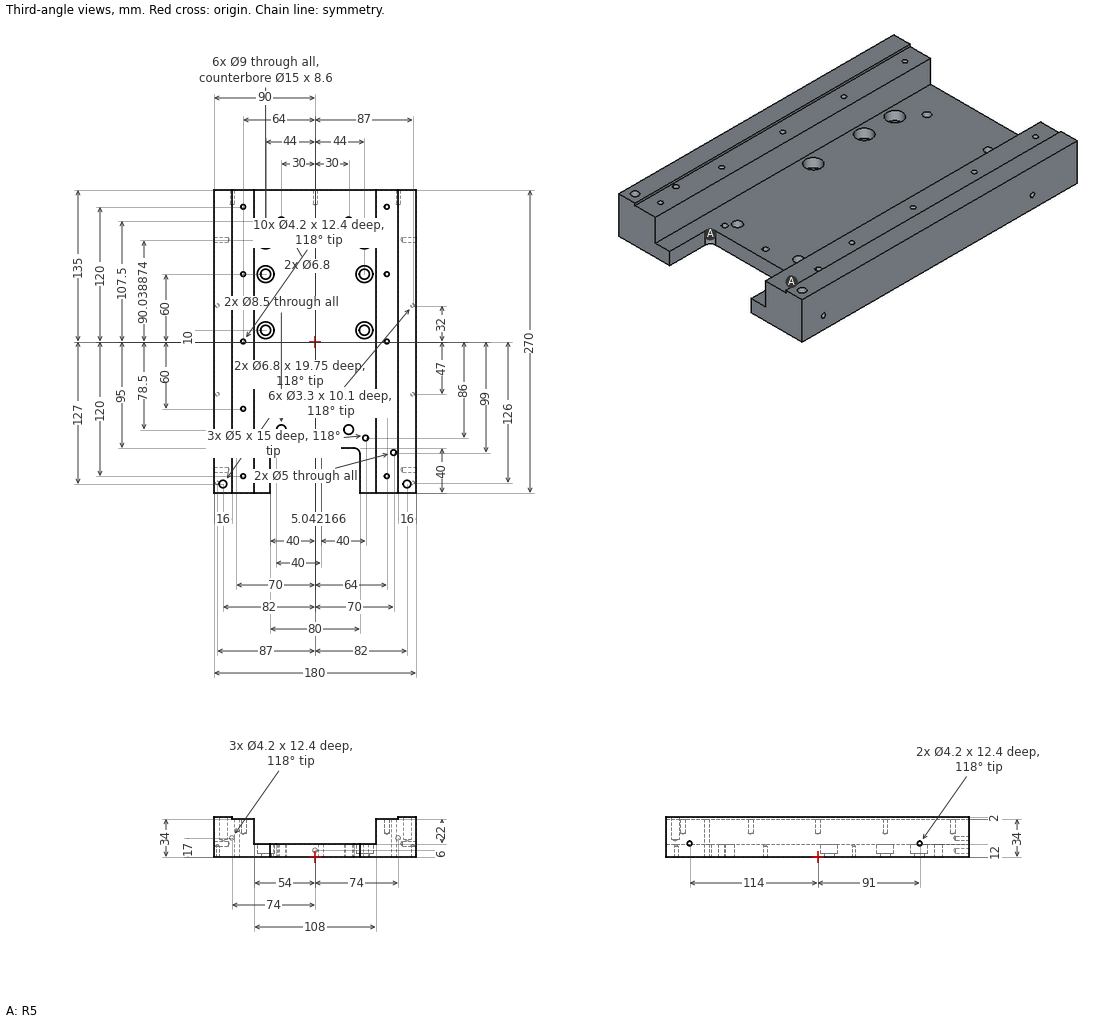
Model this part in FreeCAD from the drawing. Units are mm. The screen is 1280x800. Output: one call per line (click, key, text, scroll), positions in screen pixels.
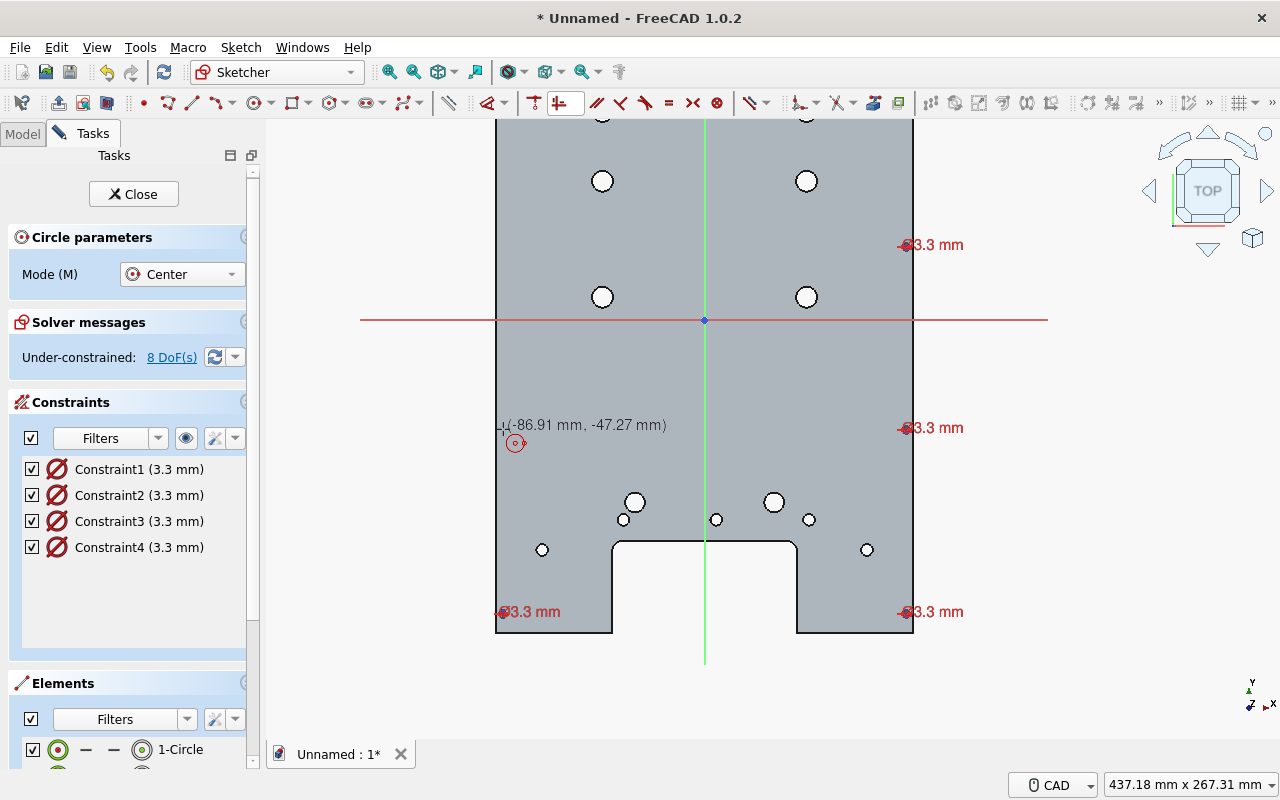
click(503, 429)
move(505, 427)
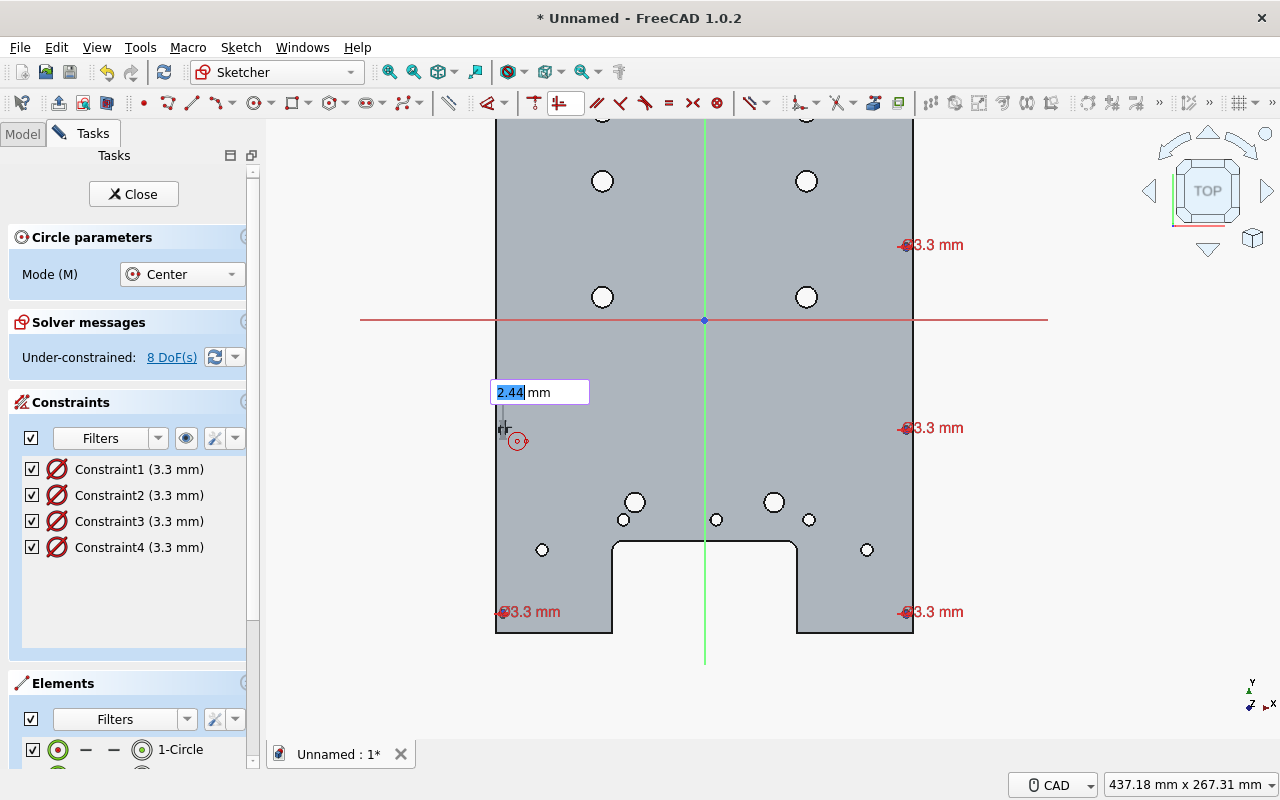
text(3.3)
key(Return)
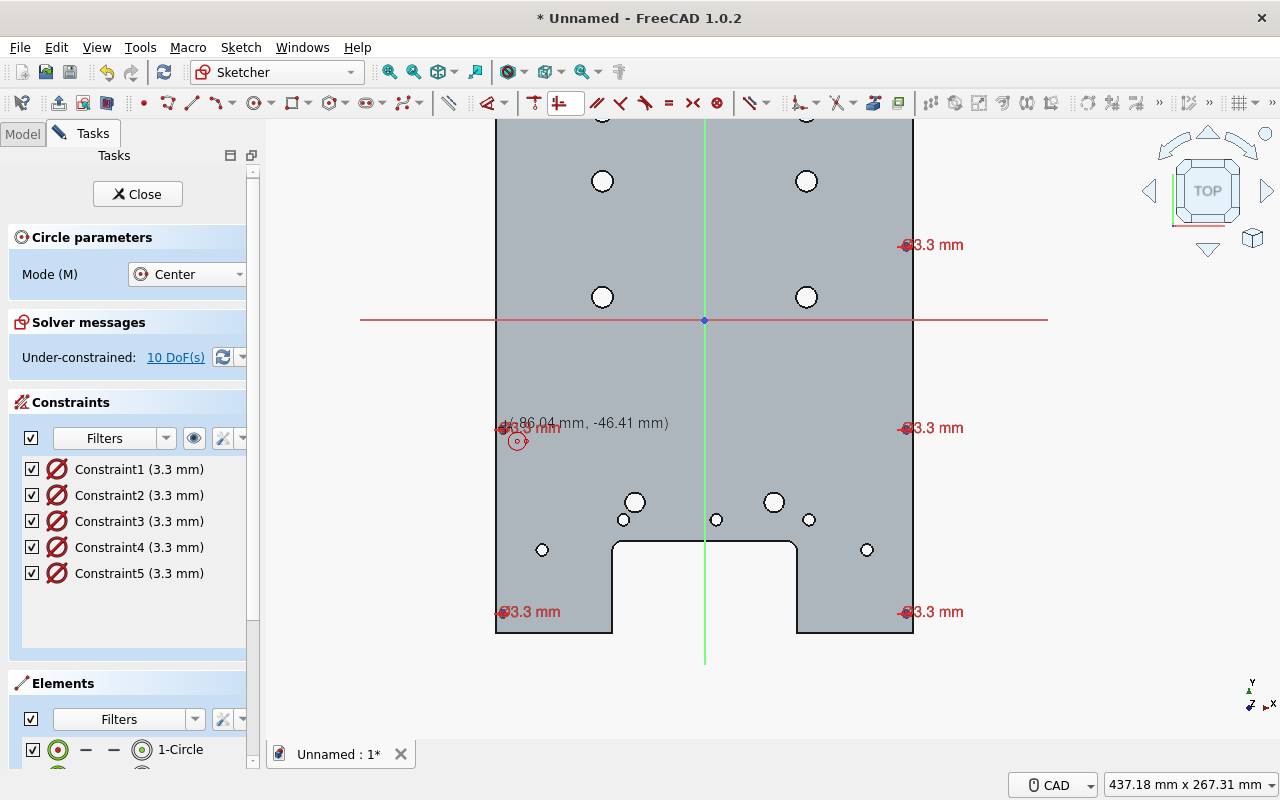
scroll(503, 246, up, 9)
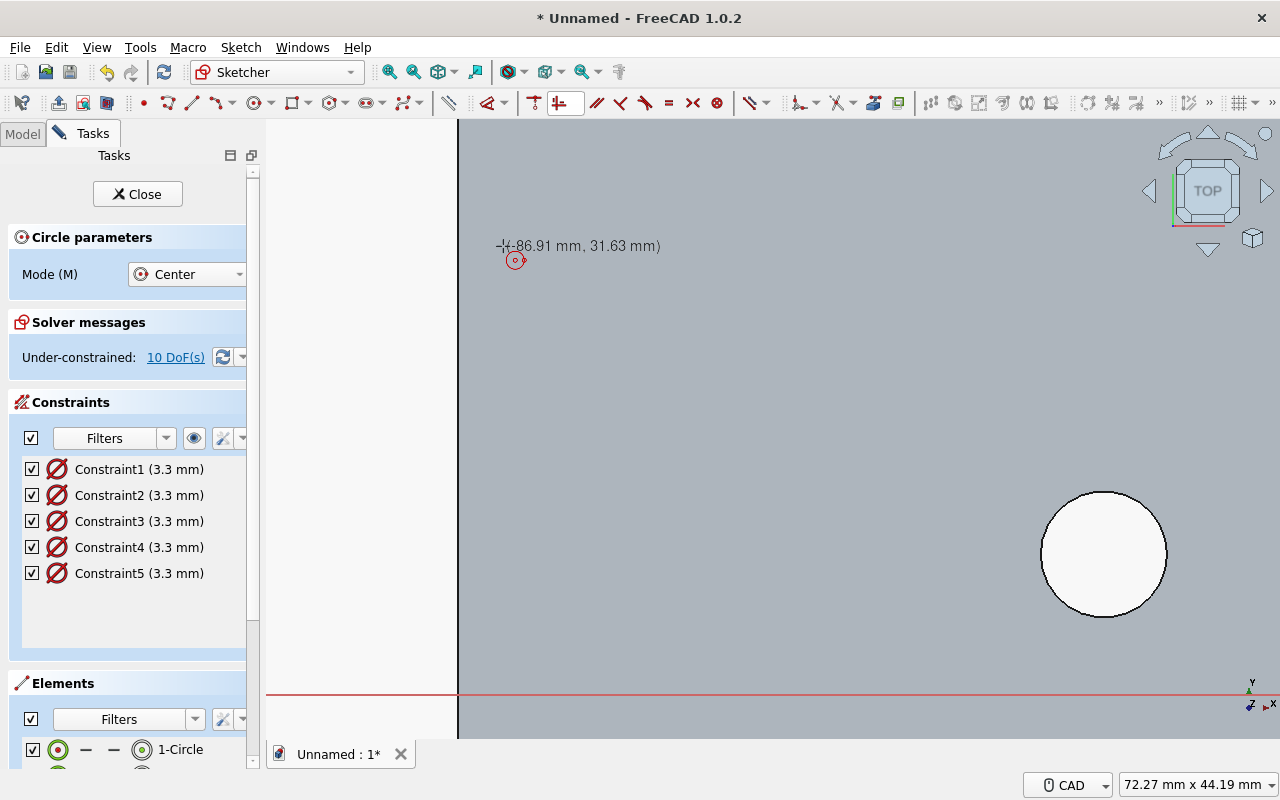
scroll(503, 246, down, 9)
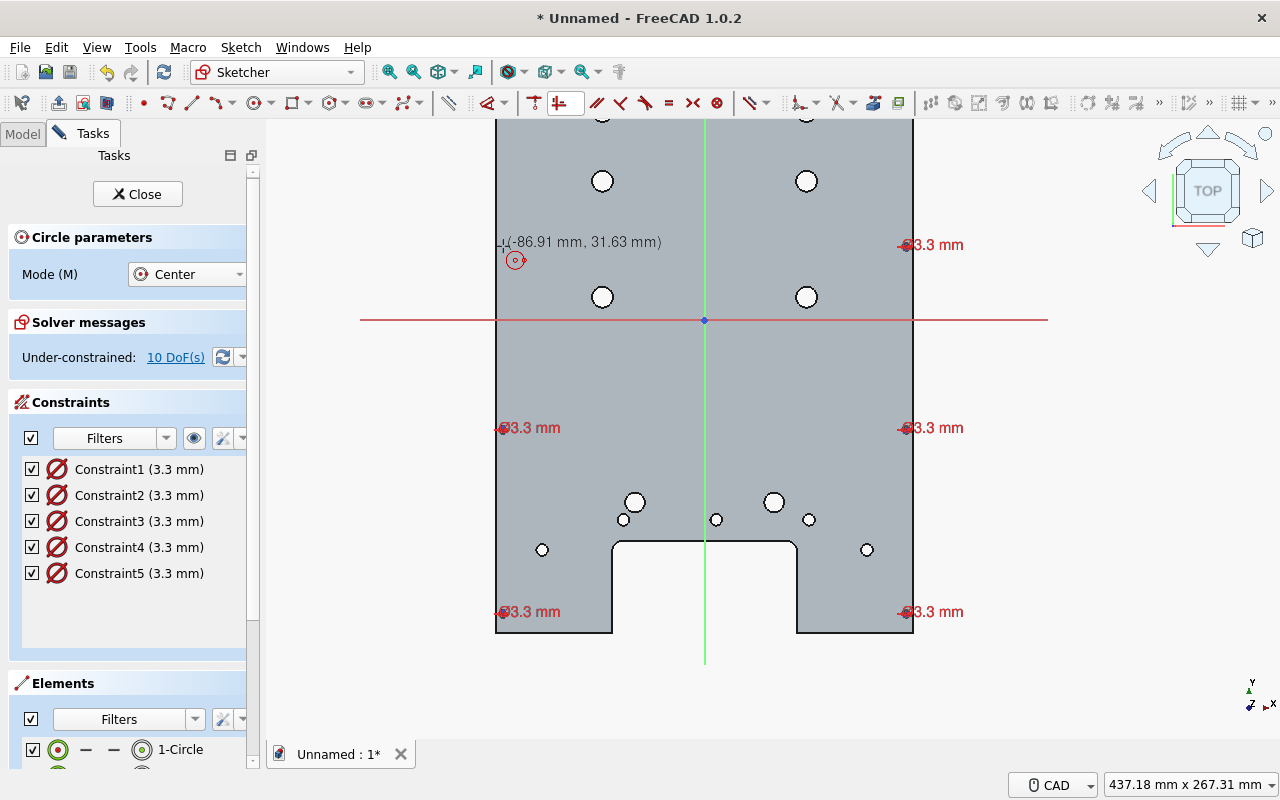
click(503, 246)
move(505, 243)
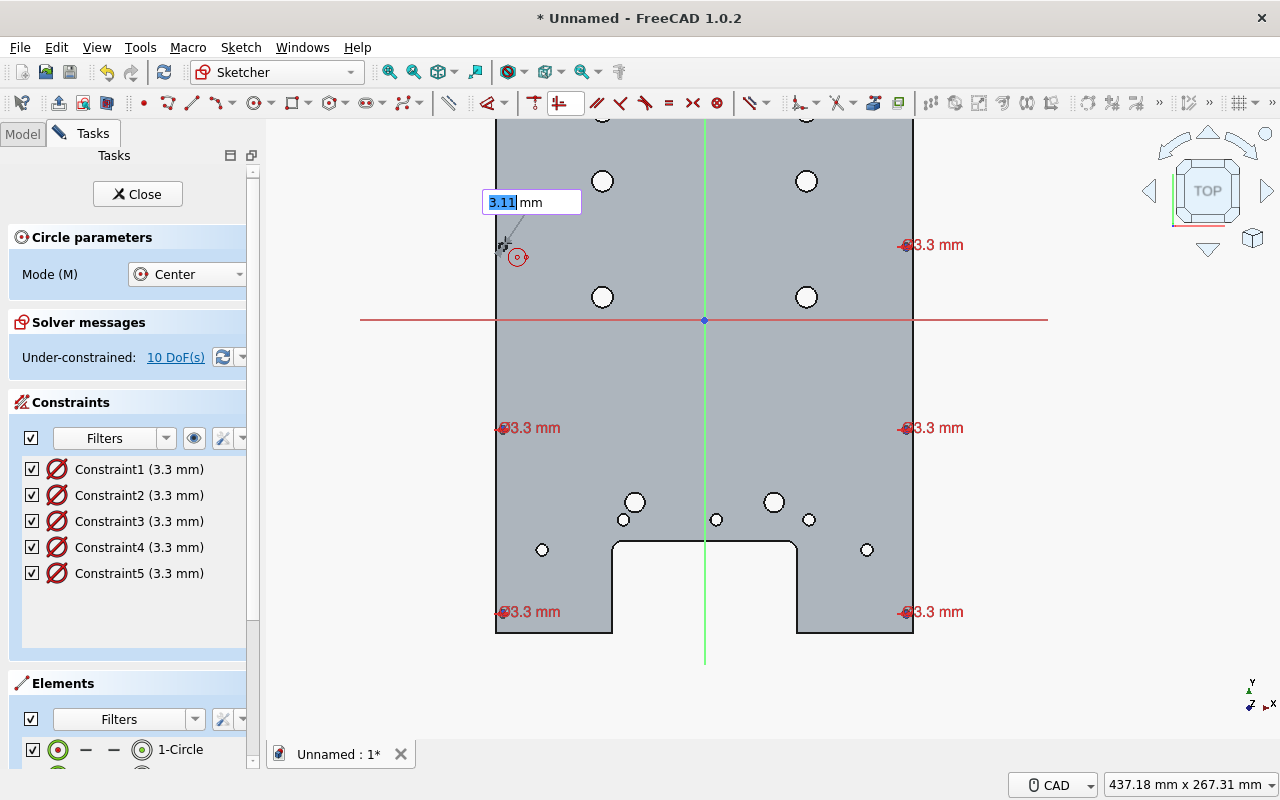
text(3.3)
key(Return)
key(Escape)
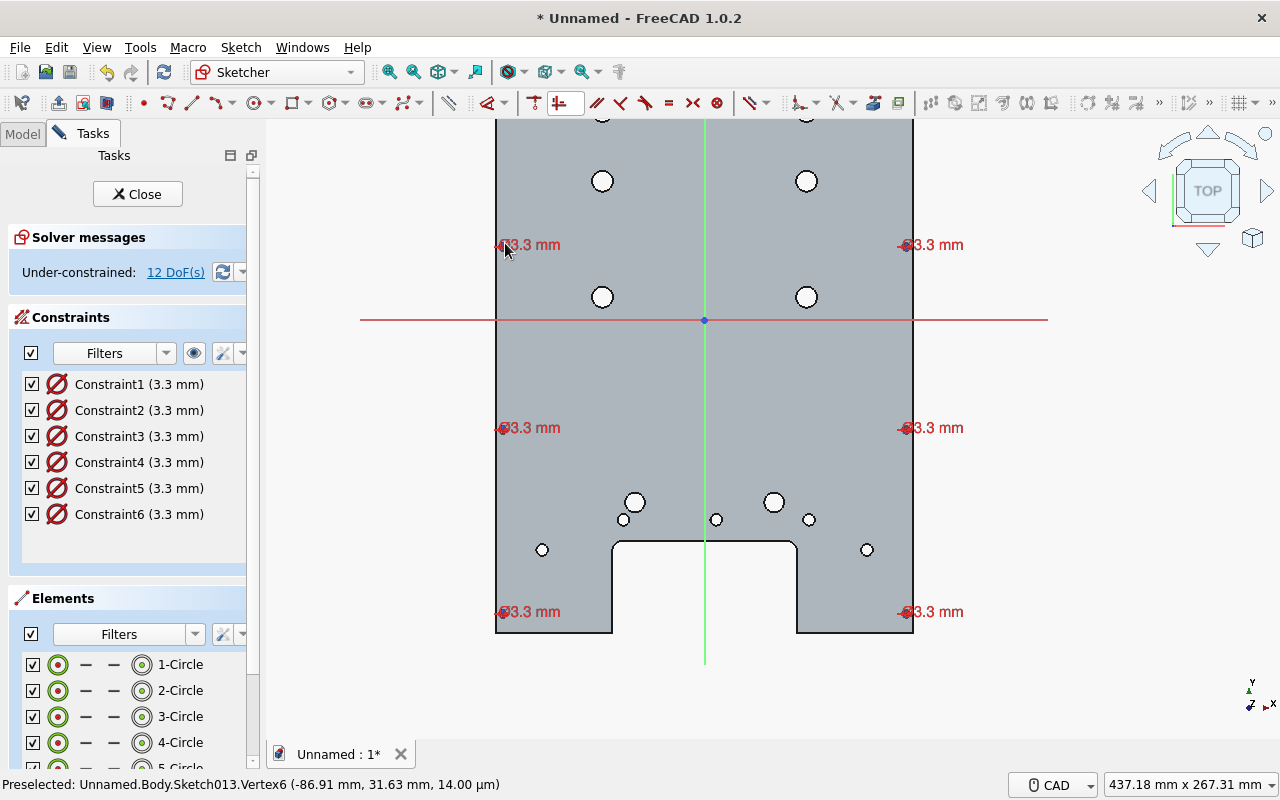
click(906, 247)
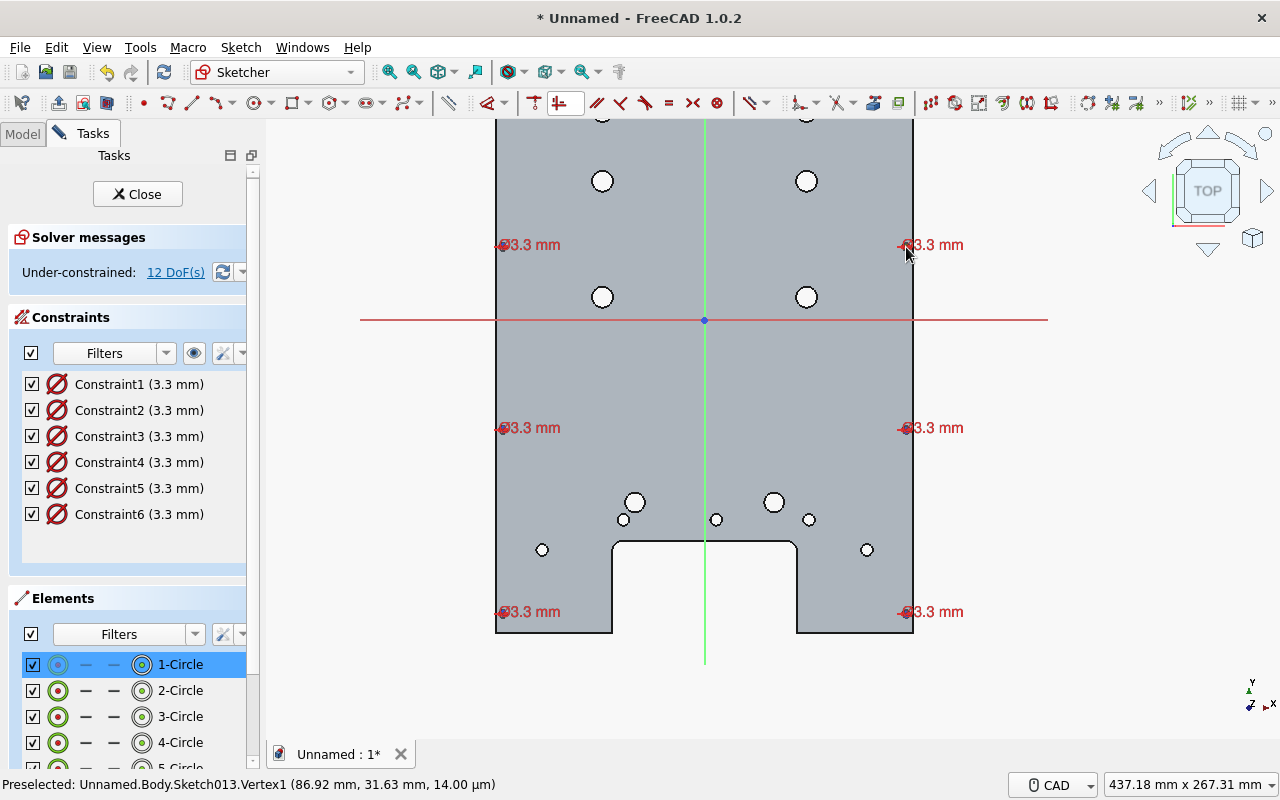
click(906, 430)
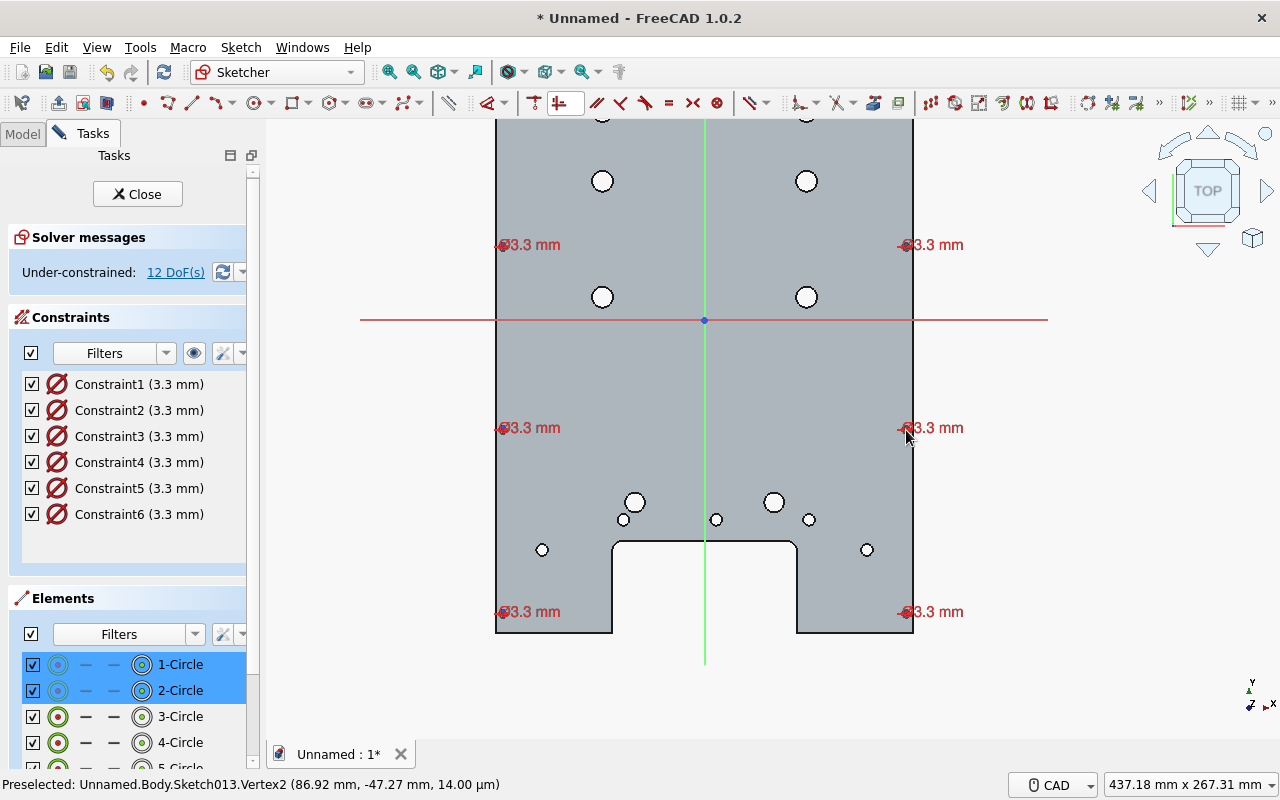
click(578, 104)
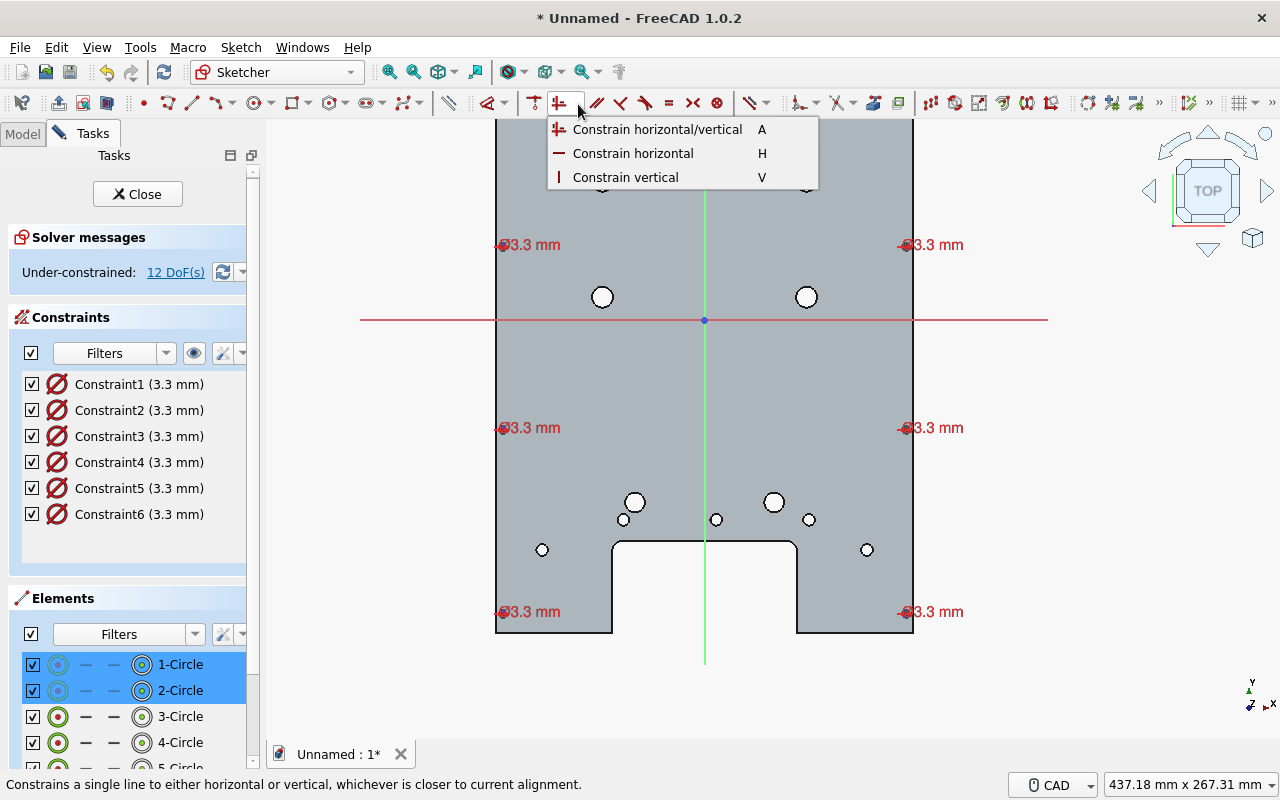
click(683, 177)